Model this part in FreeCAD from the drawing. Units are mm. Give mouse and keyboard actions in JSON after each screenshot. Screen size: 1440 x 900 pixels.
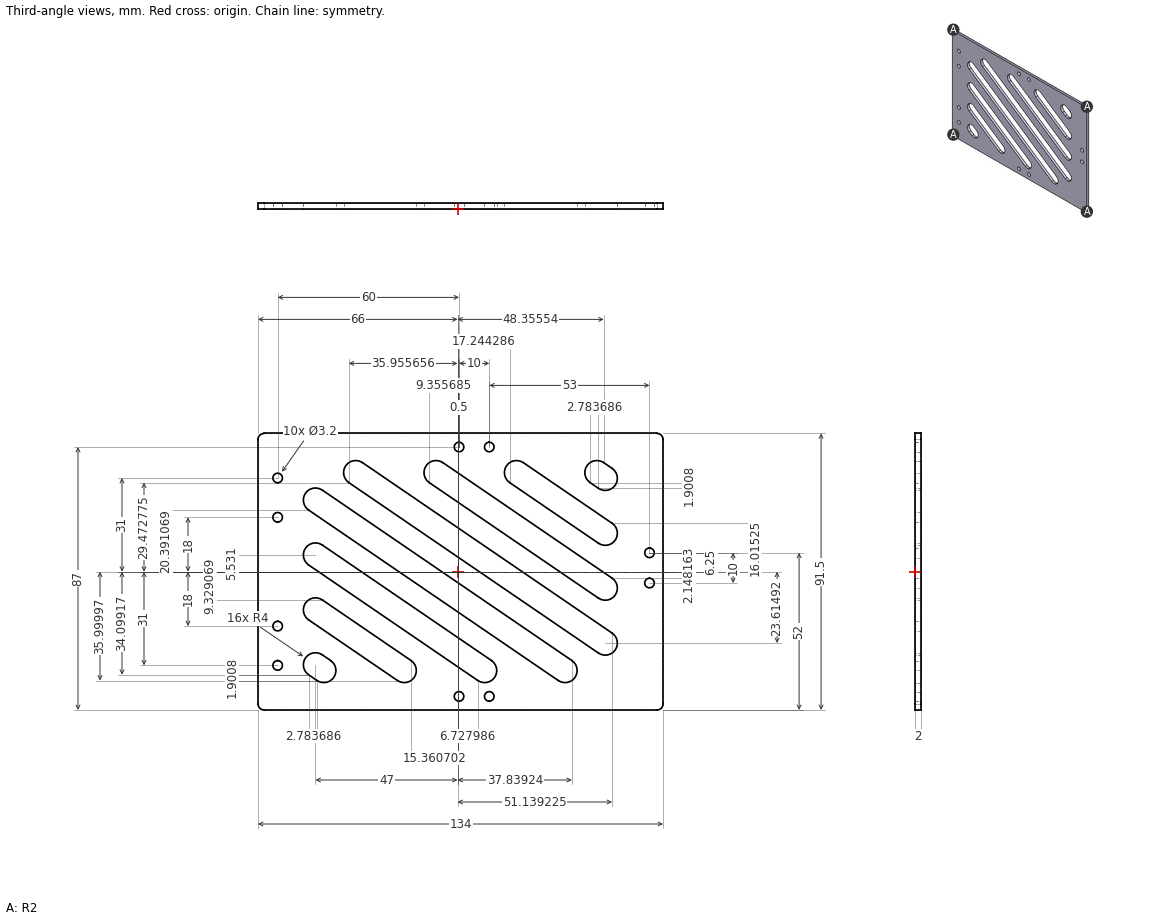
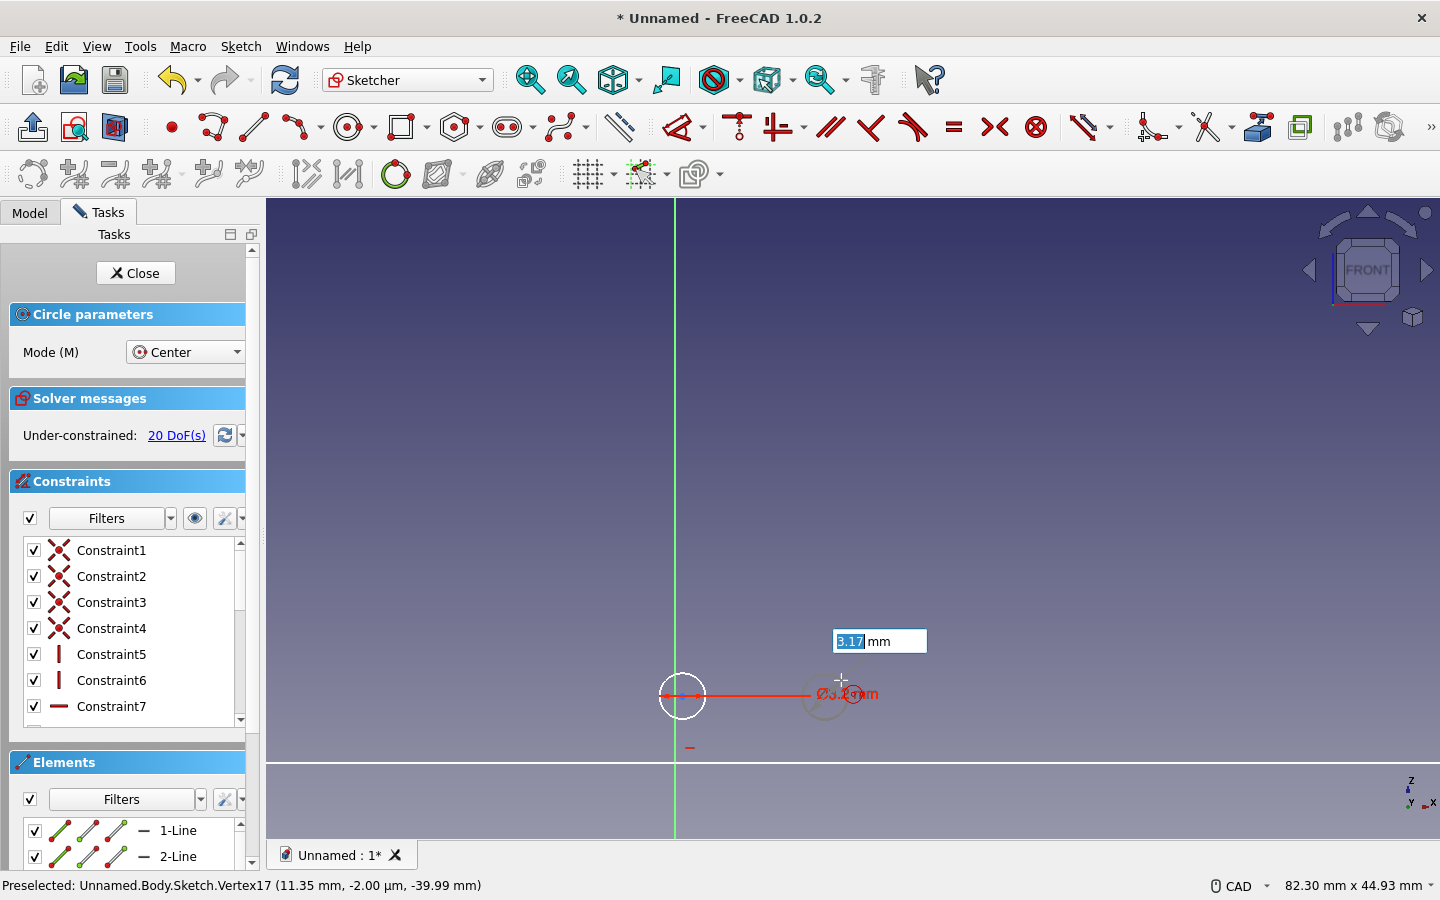
{"action": "type", "text": "3.2"}
{"action": "key", "text": "Return"}
{"action": "key", "text": "Escape"}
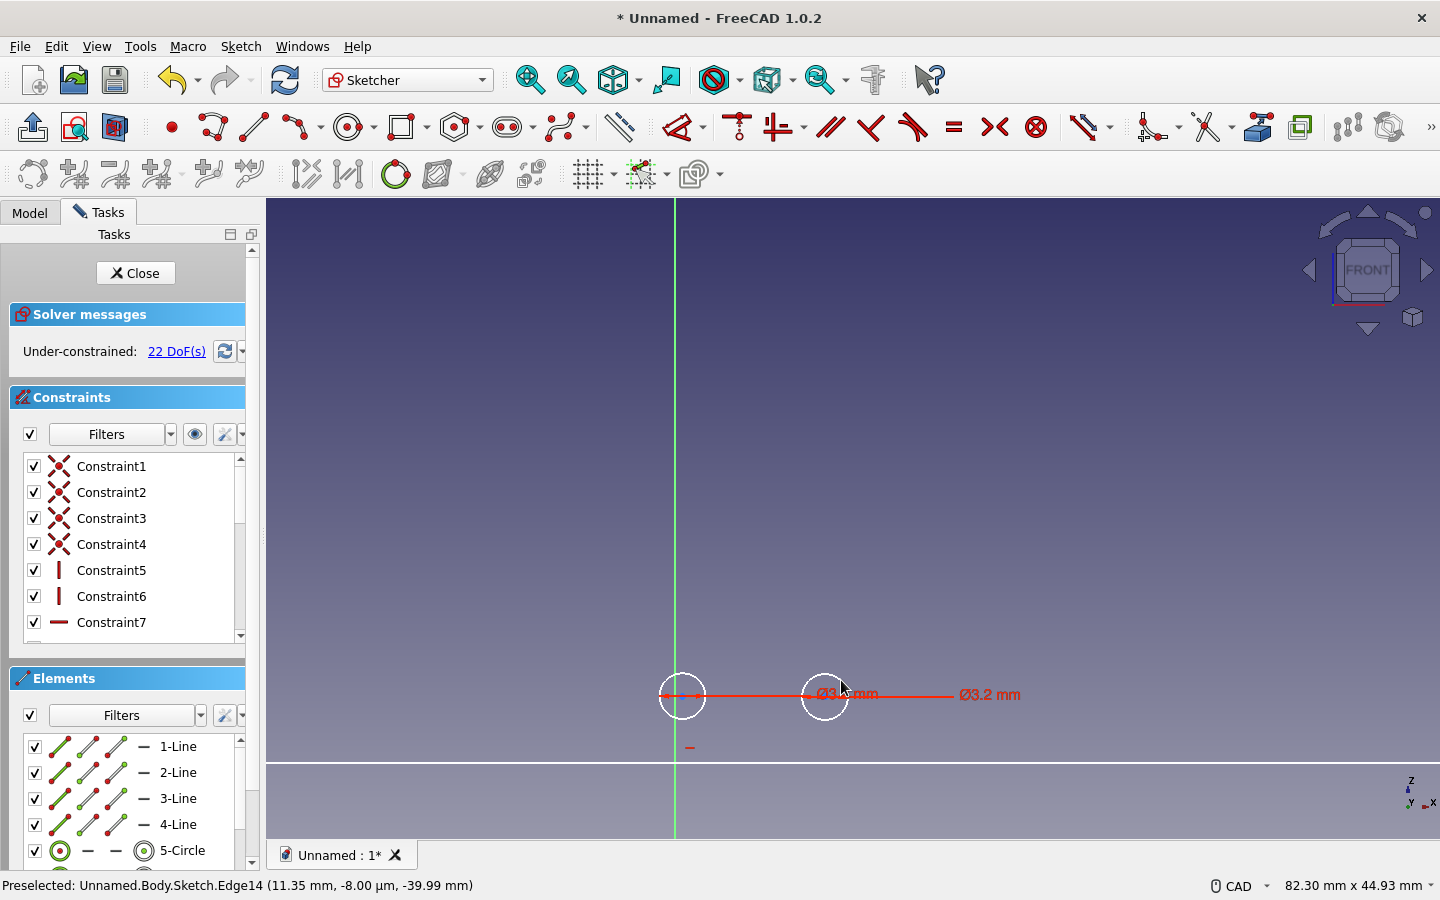
{"action": "scroll", "coordinate": [825, 696], "scroll_direction": "down", "scroll_amount": 6}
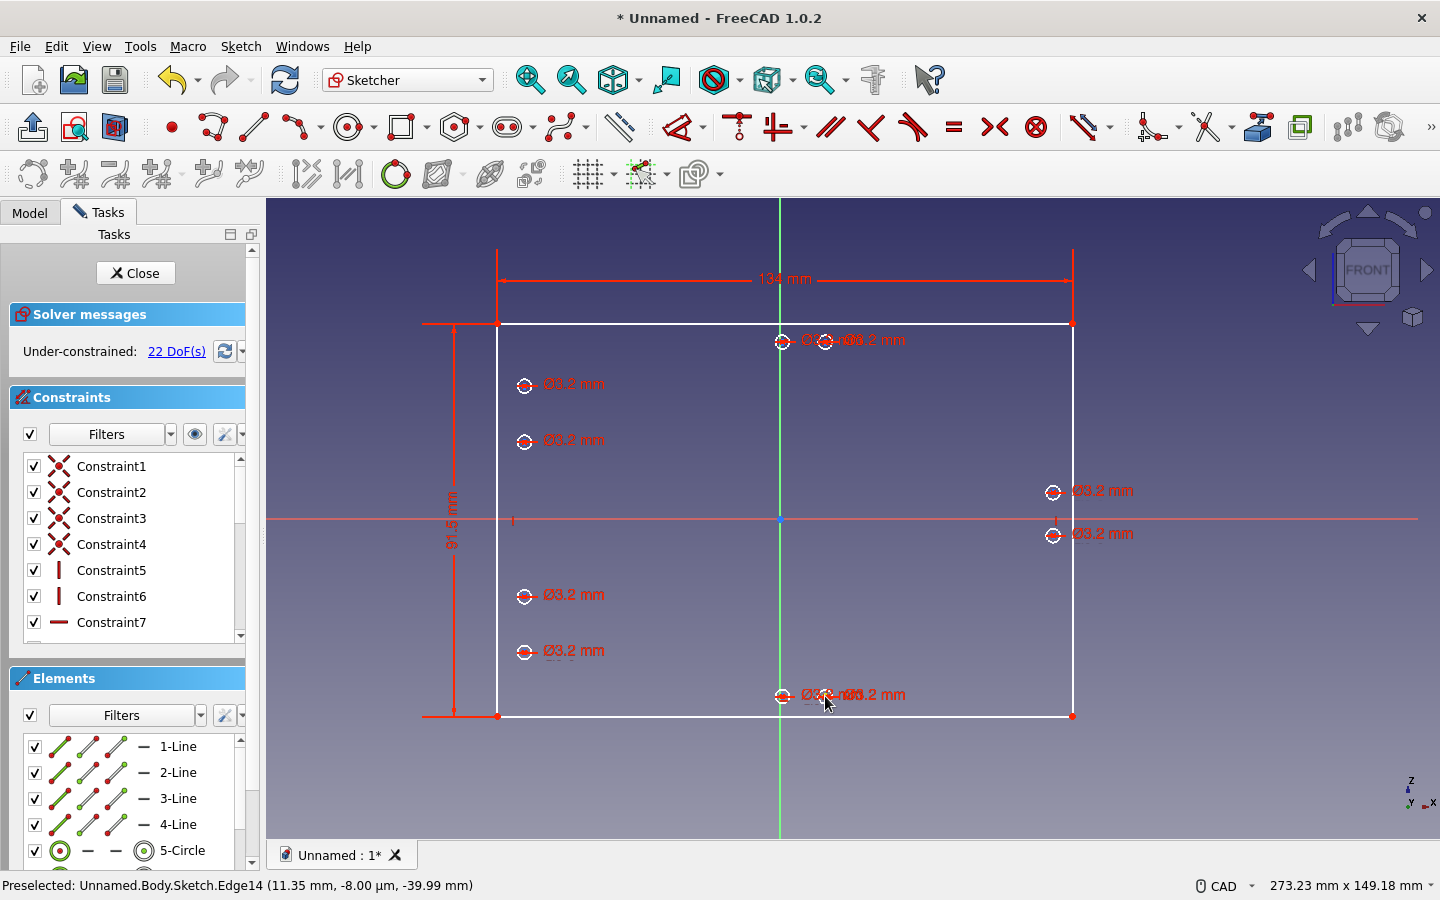
{"action": "left_click", "coordinate": [525, 386]}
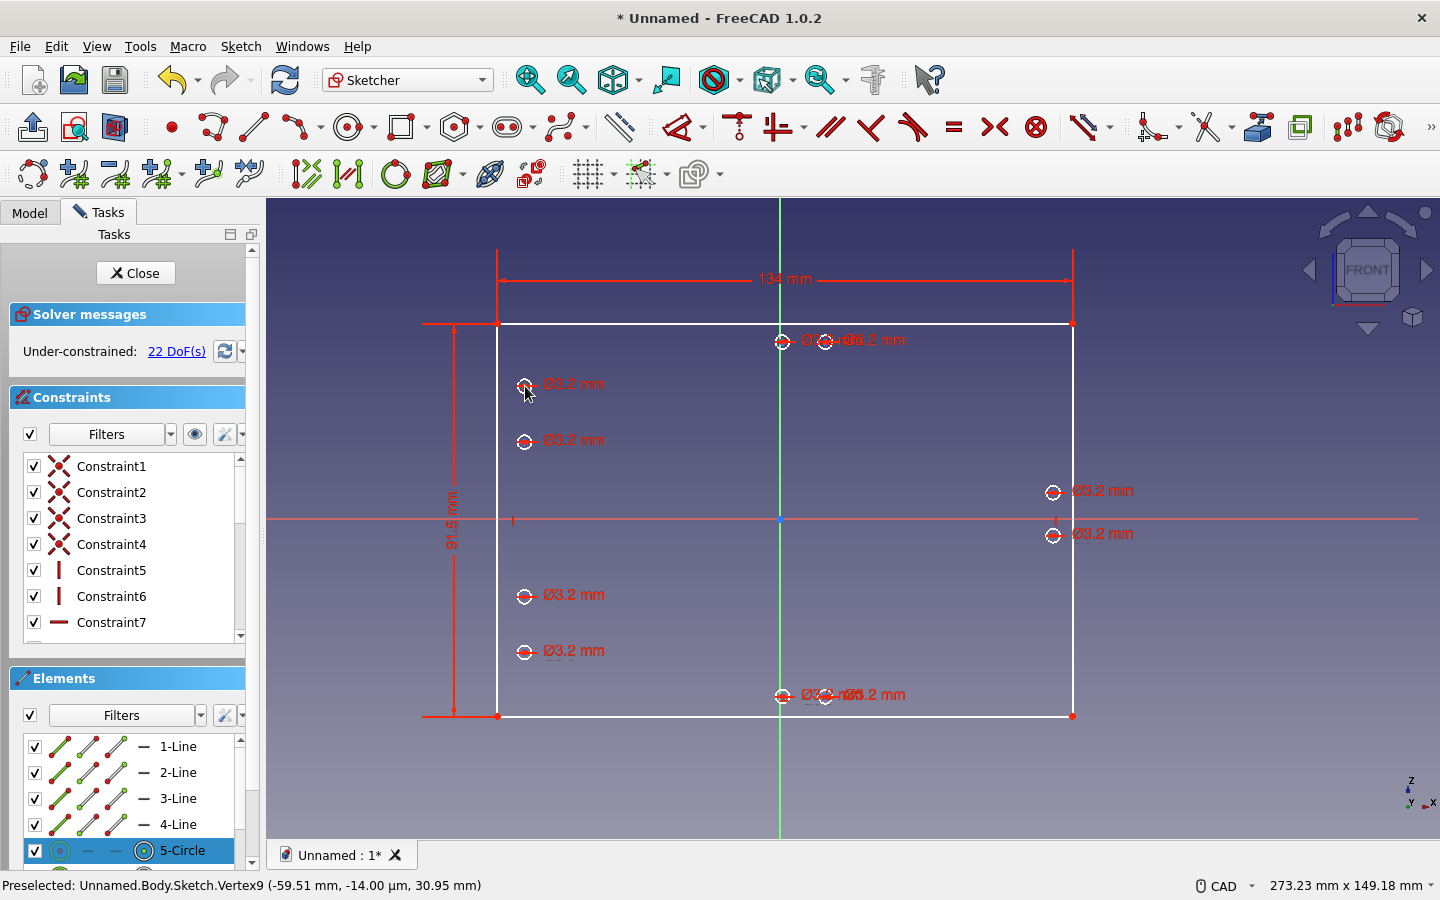
{"action": "left_click", "coordinate": [525, 442]}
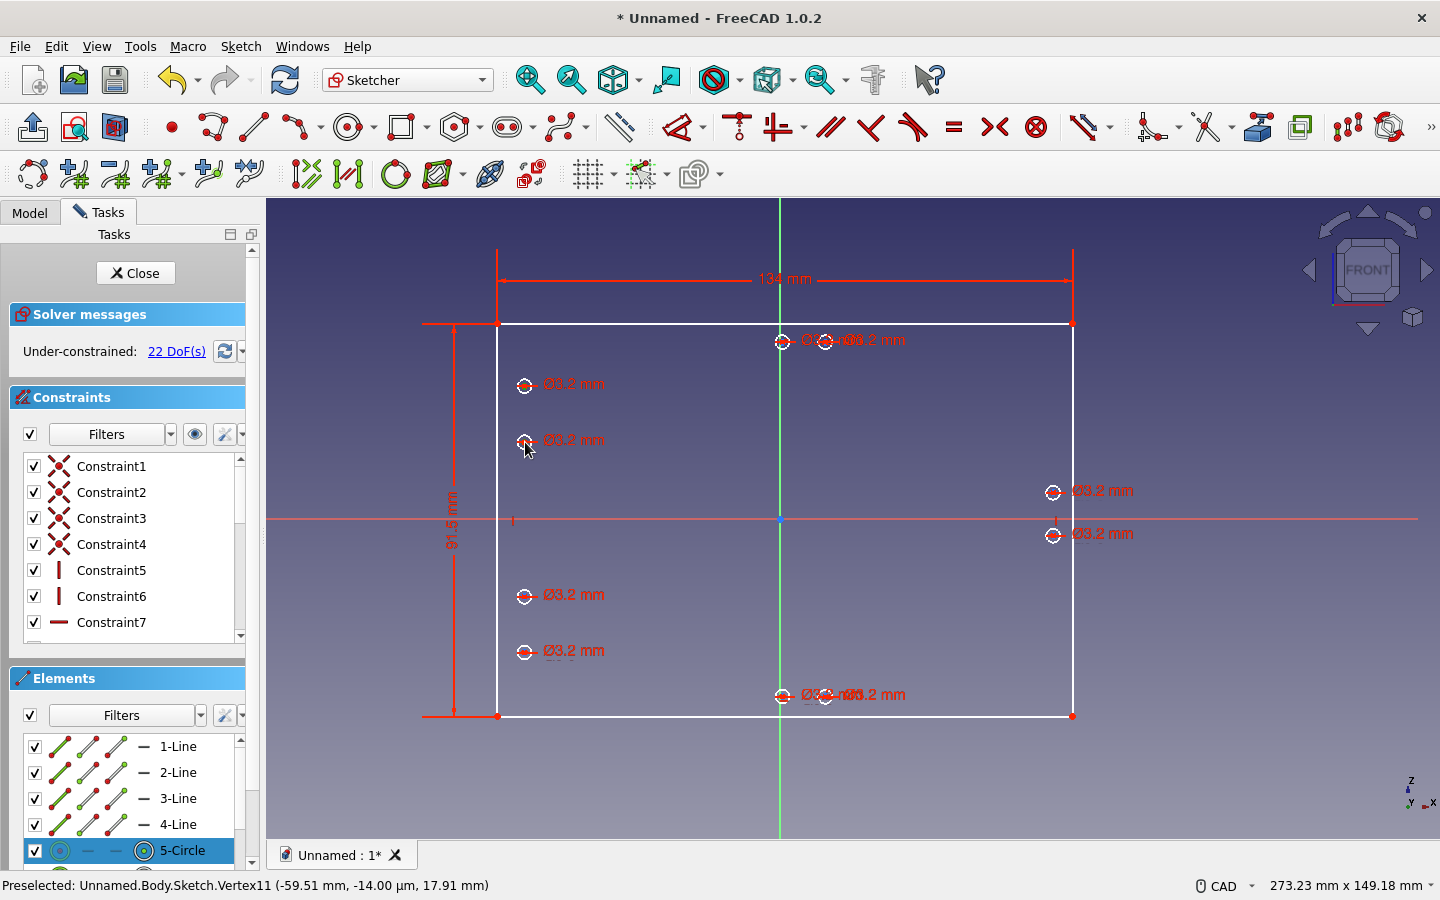
{"action": "left_click", "coordinate": [804, 128]}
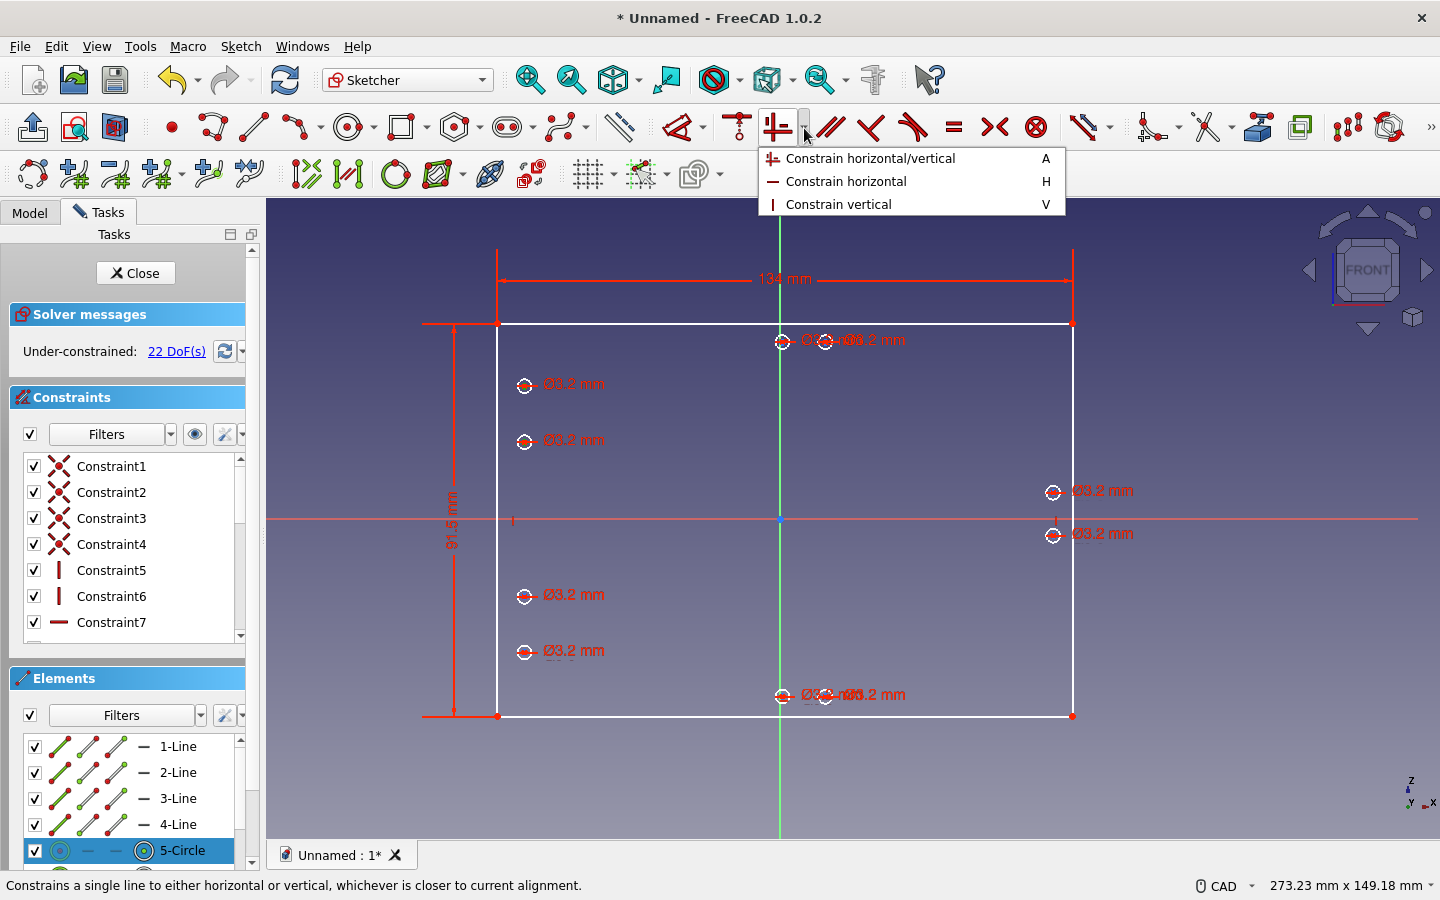
{"action": "left_click", "coordinate": [912, 204]}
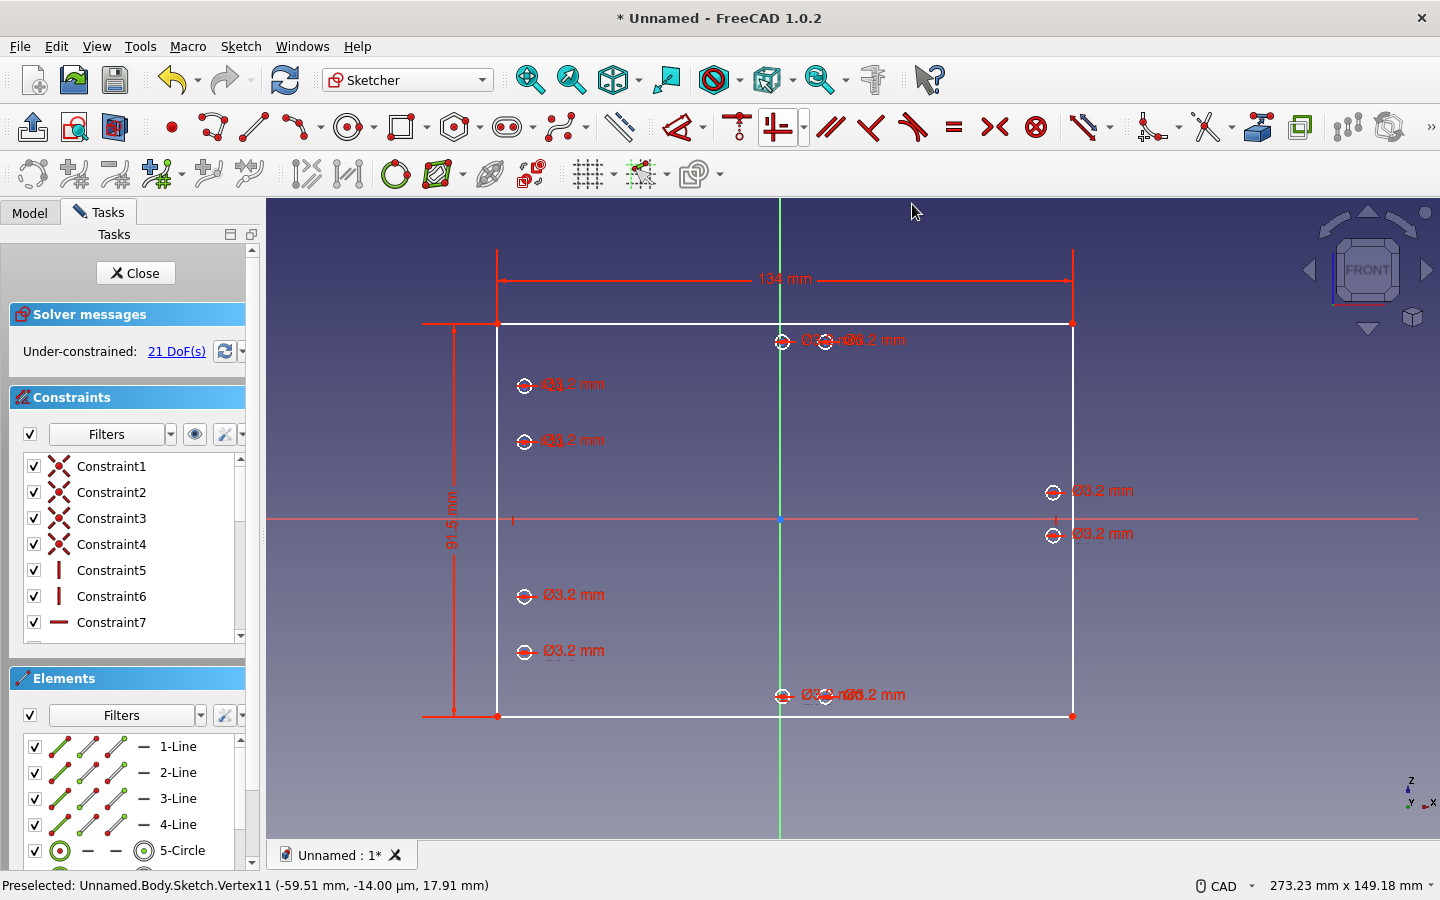
{"action": "left_click", "coordinate": [782, 342]}